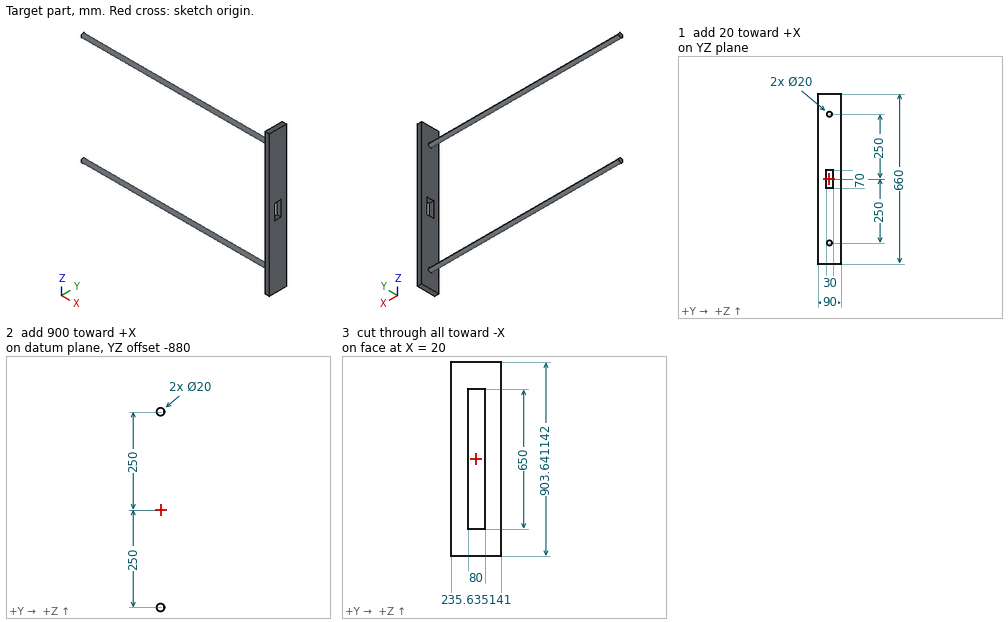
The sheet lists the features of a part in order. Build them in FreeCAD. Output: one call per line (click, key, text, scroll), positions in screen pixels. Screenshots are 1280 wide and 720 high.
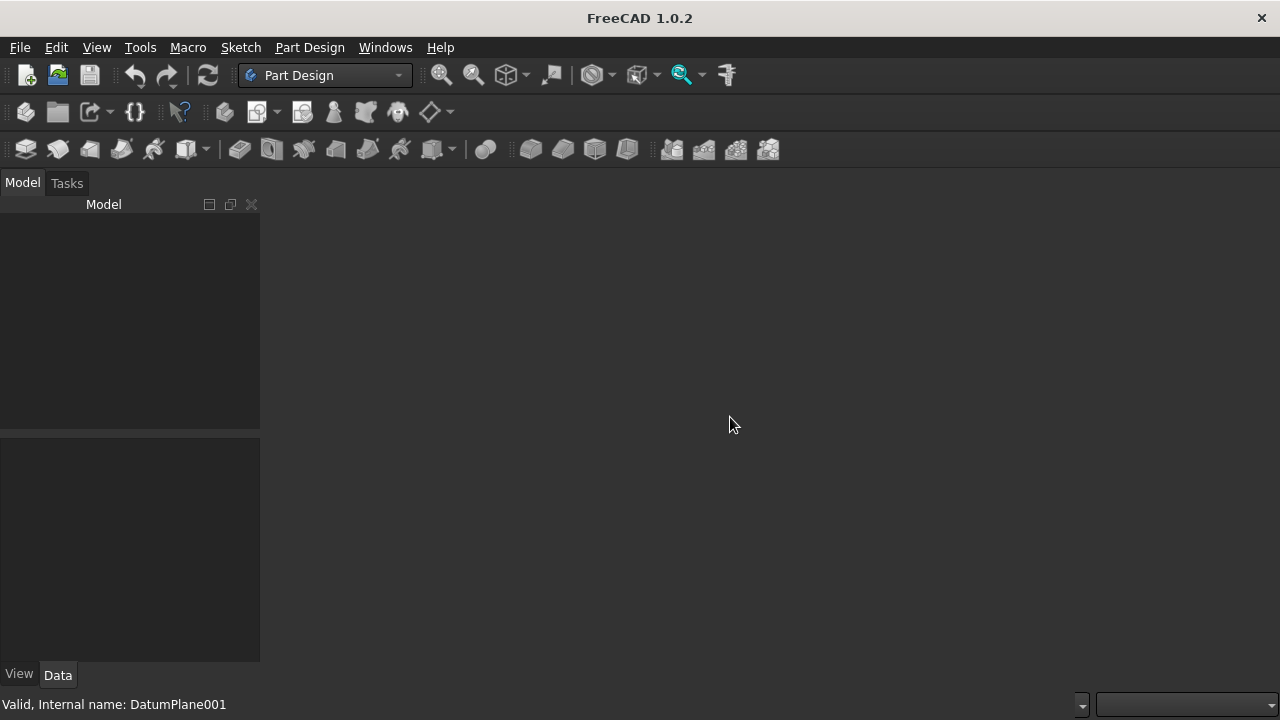
click(26, 76)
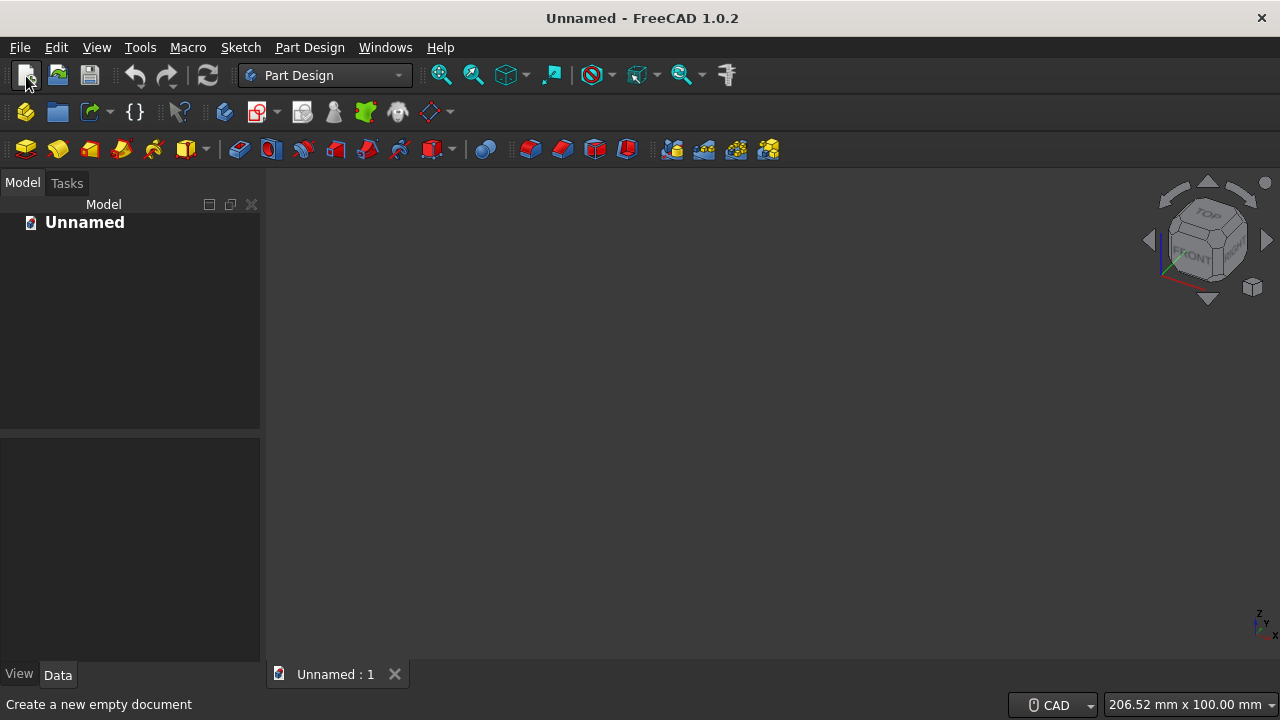
click(258, 112)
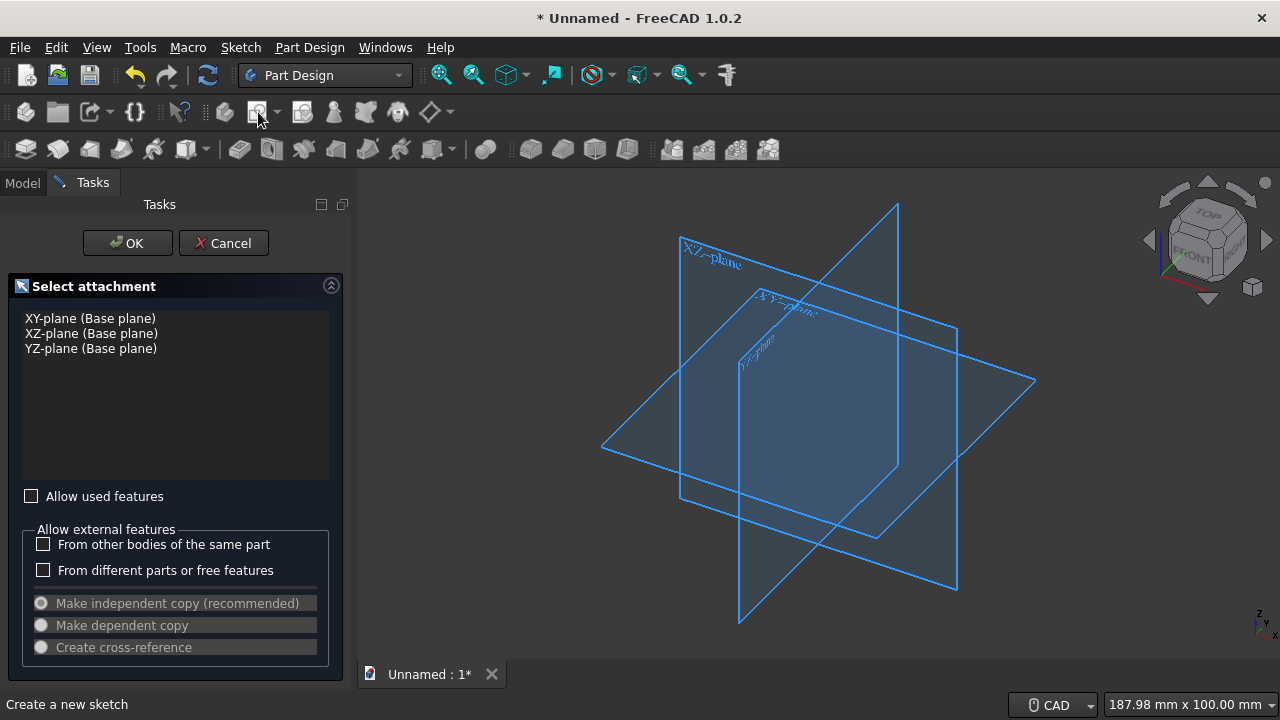
click(82, 348)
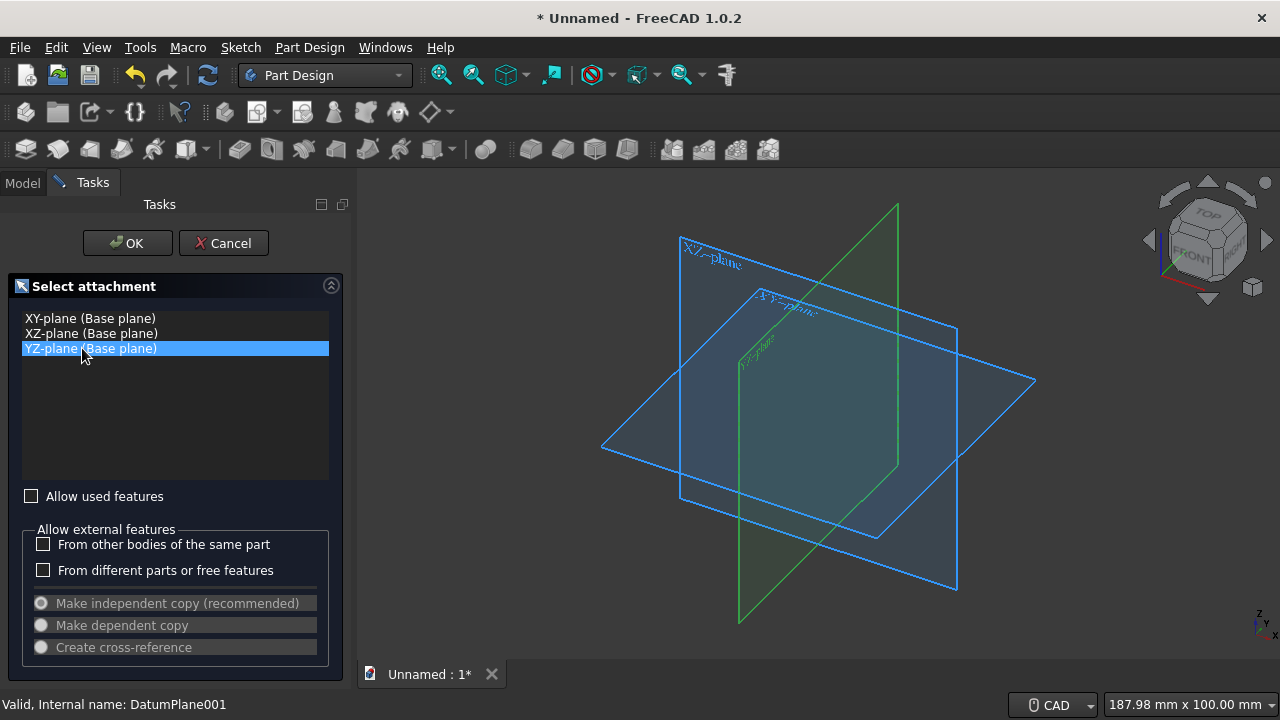
click(128, 243)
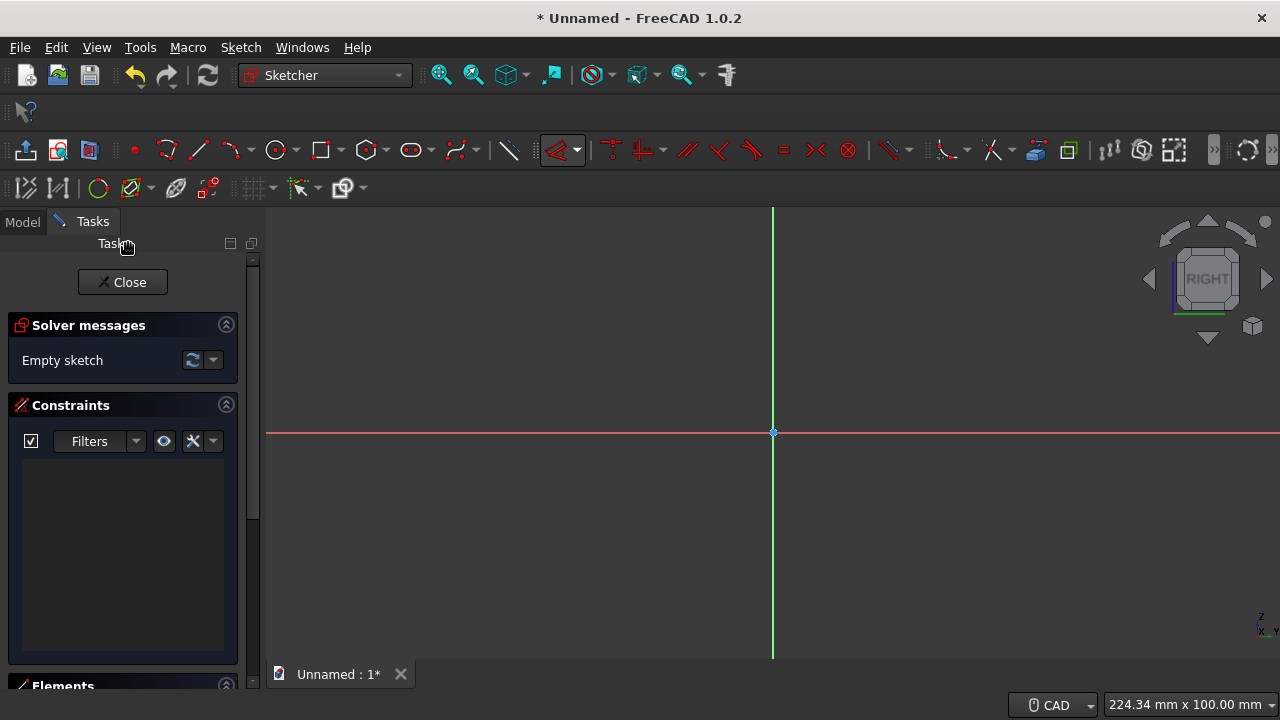
scroll(698, 433, down, 12)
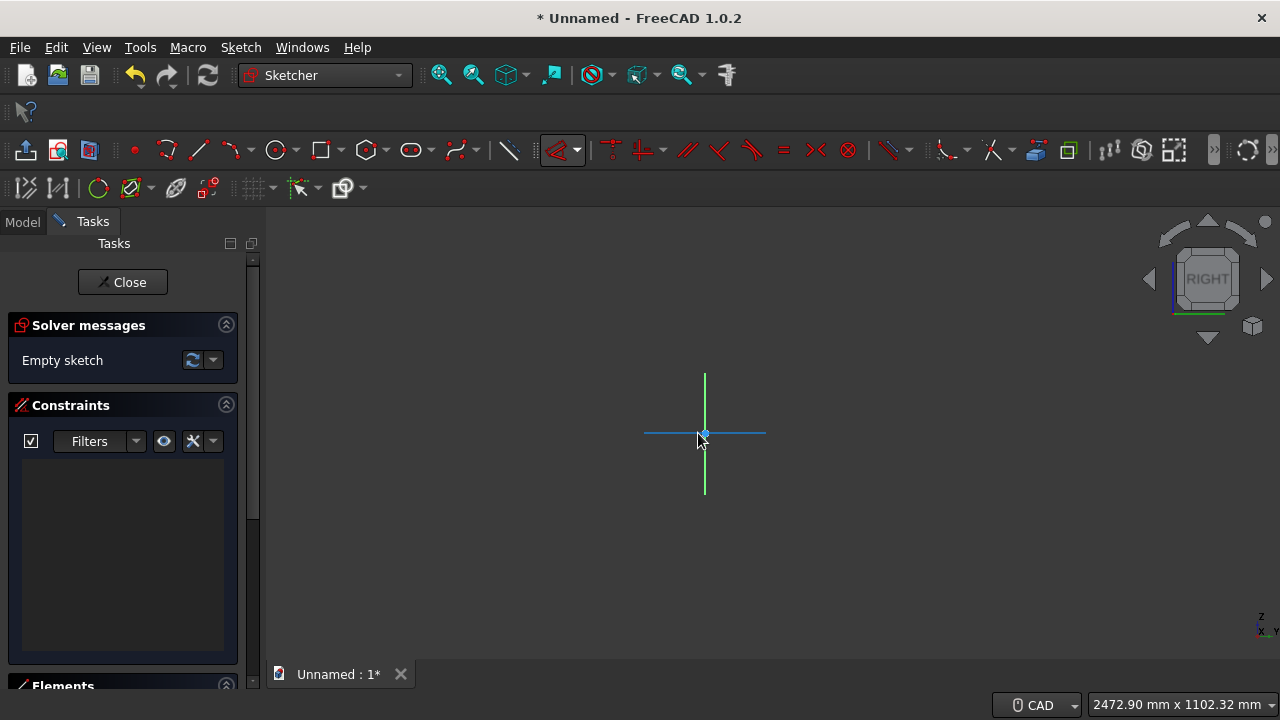
key(g)
key(v)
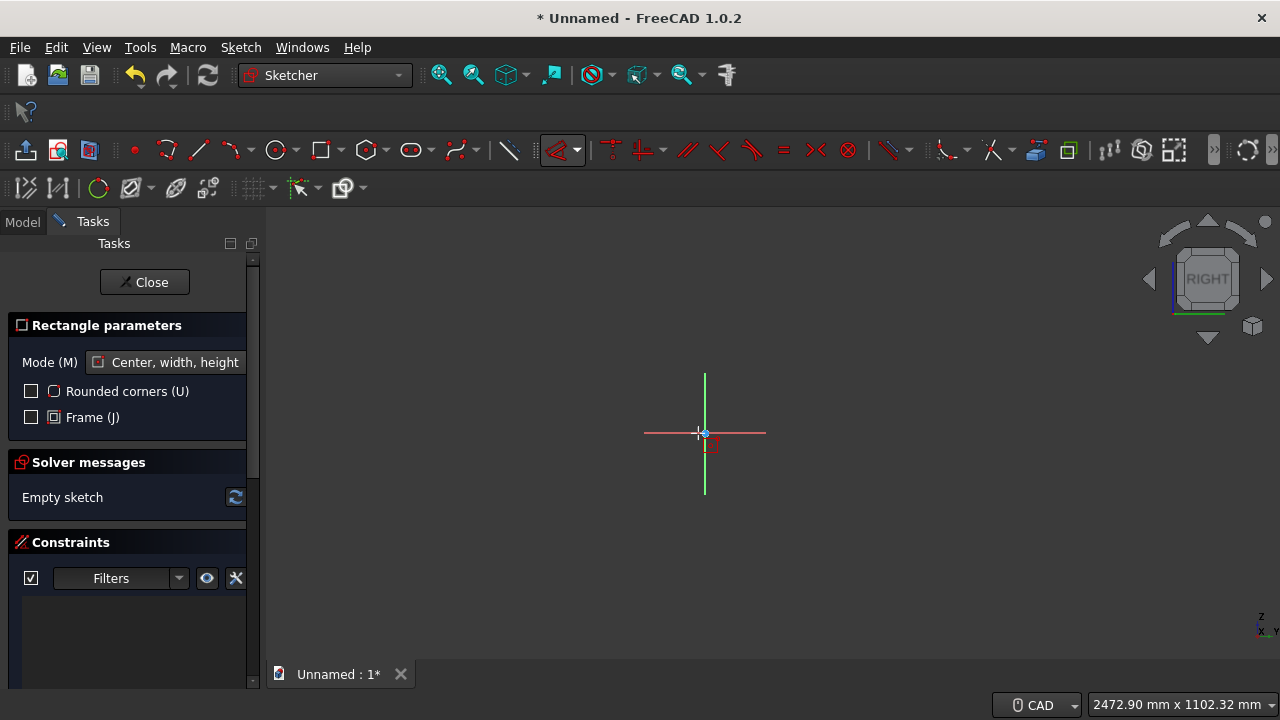
click(705, 433)
click(724, 298)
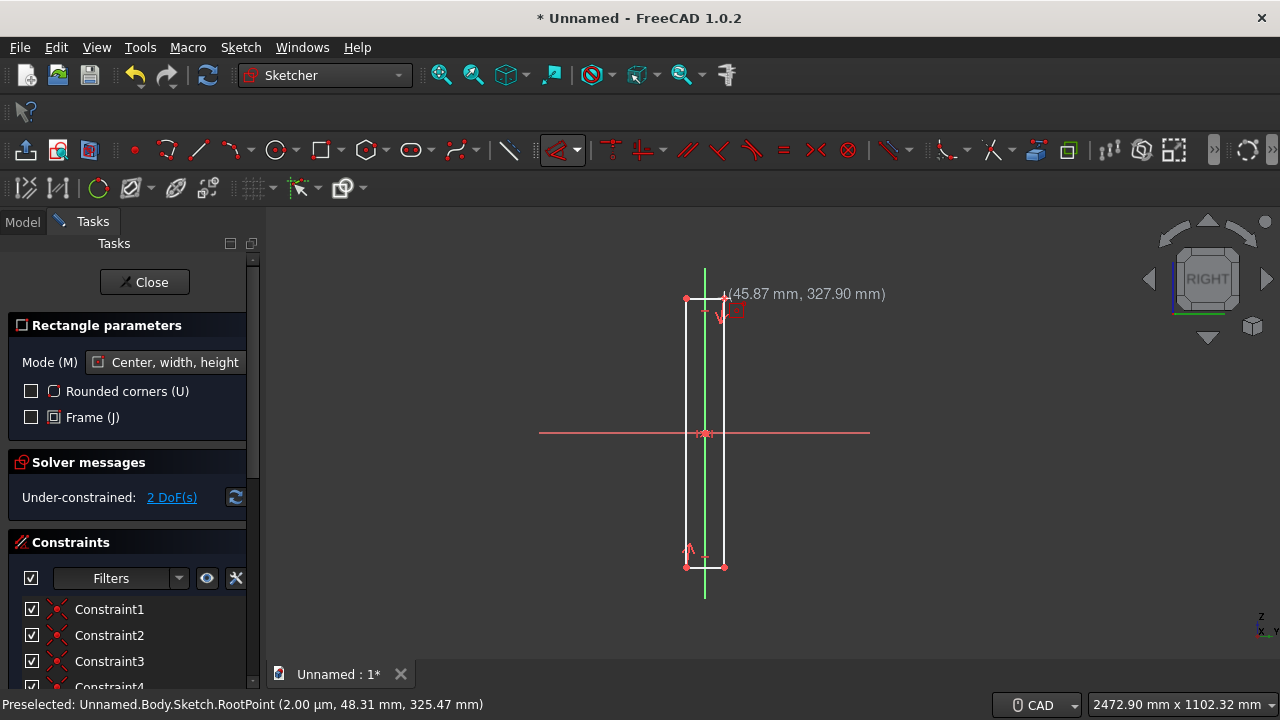
scroll(705, 433, up, 5)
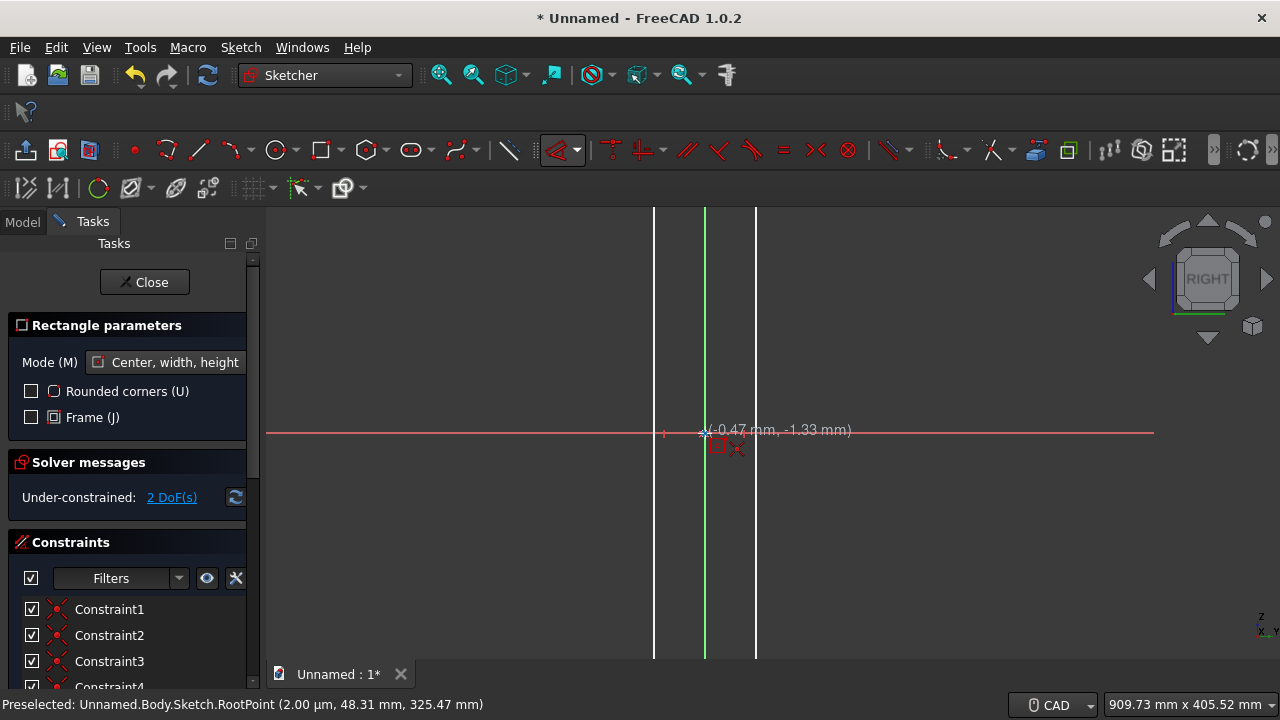
click(705, 433)
click(721, 394)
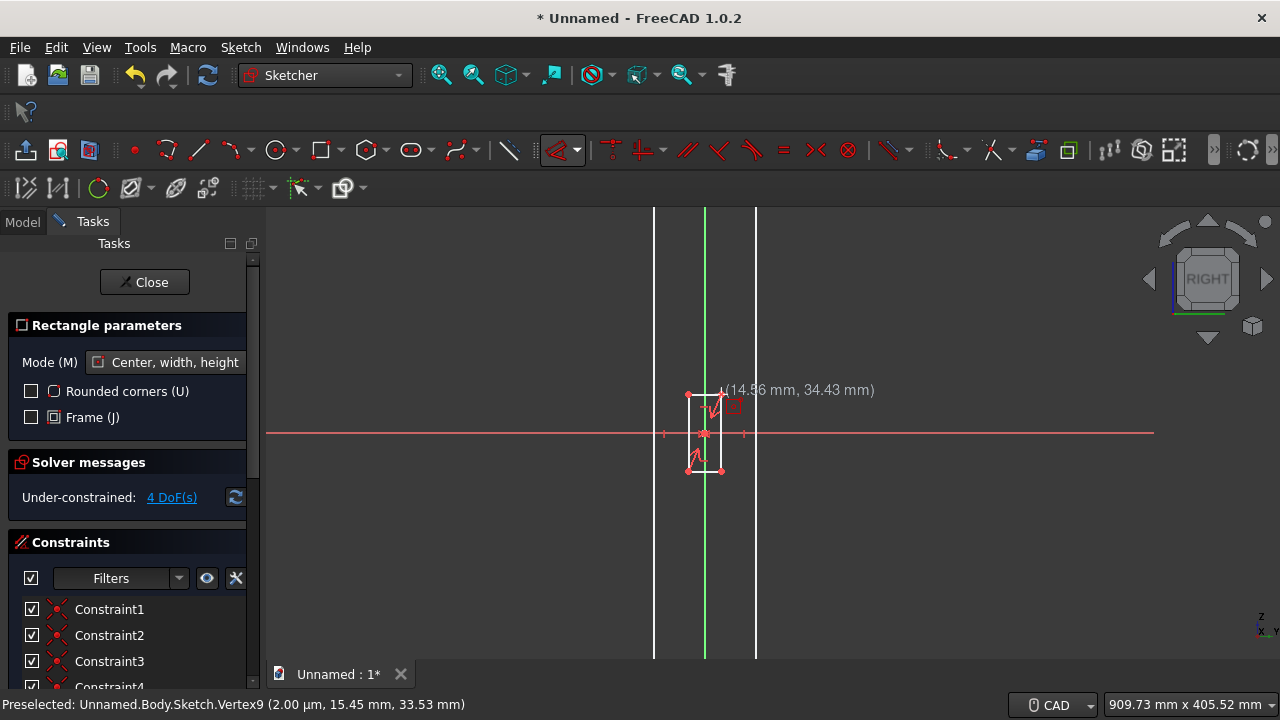
key(g)
key(c)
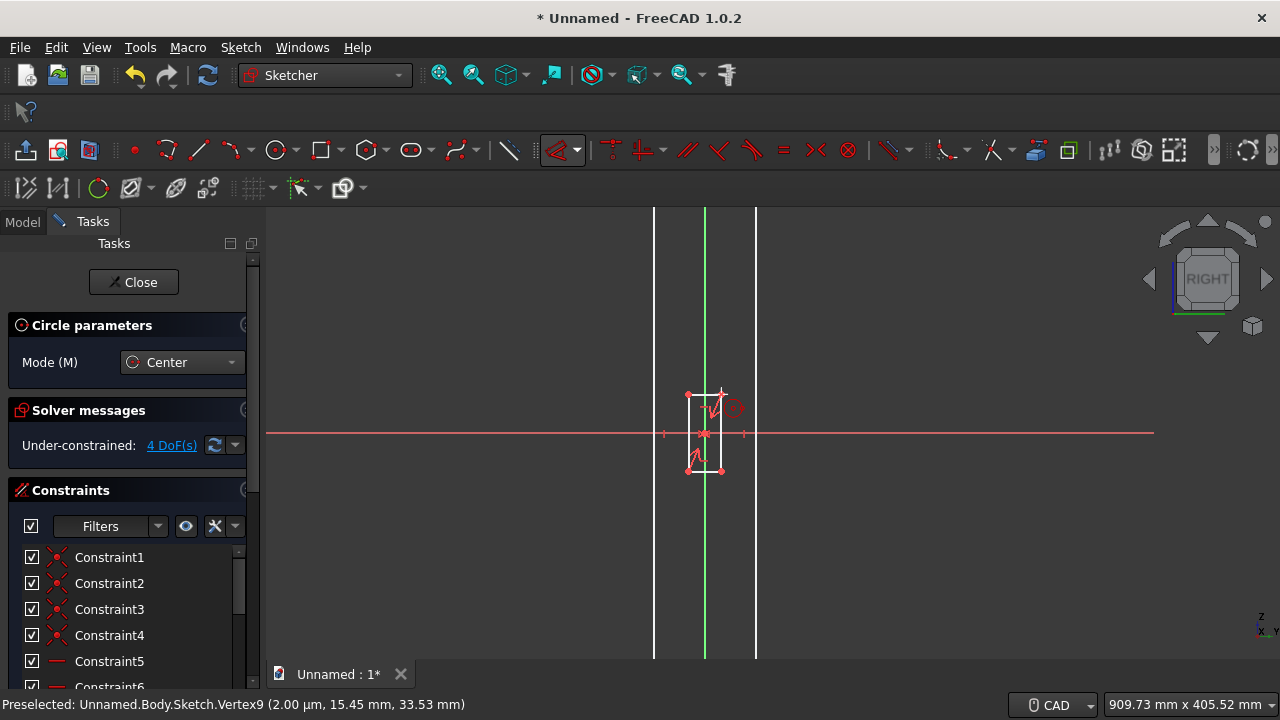
scroll(704, 433, down, 5)